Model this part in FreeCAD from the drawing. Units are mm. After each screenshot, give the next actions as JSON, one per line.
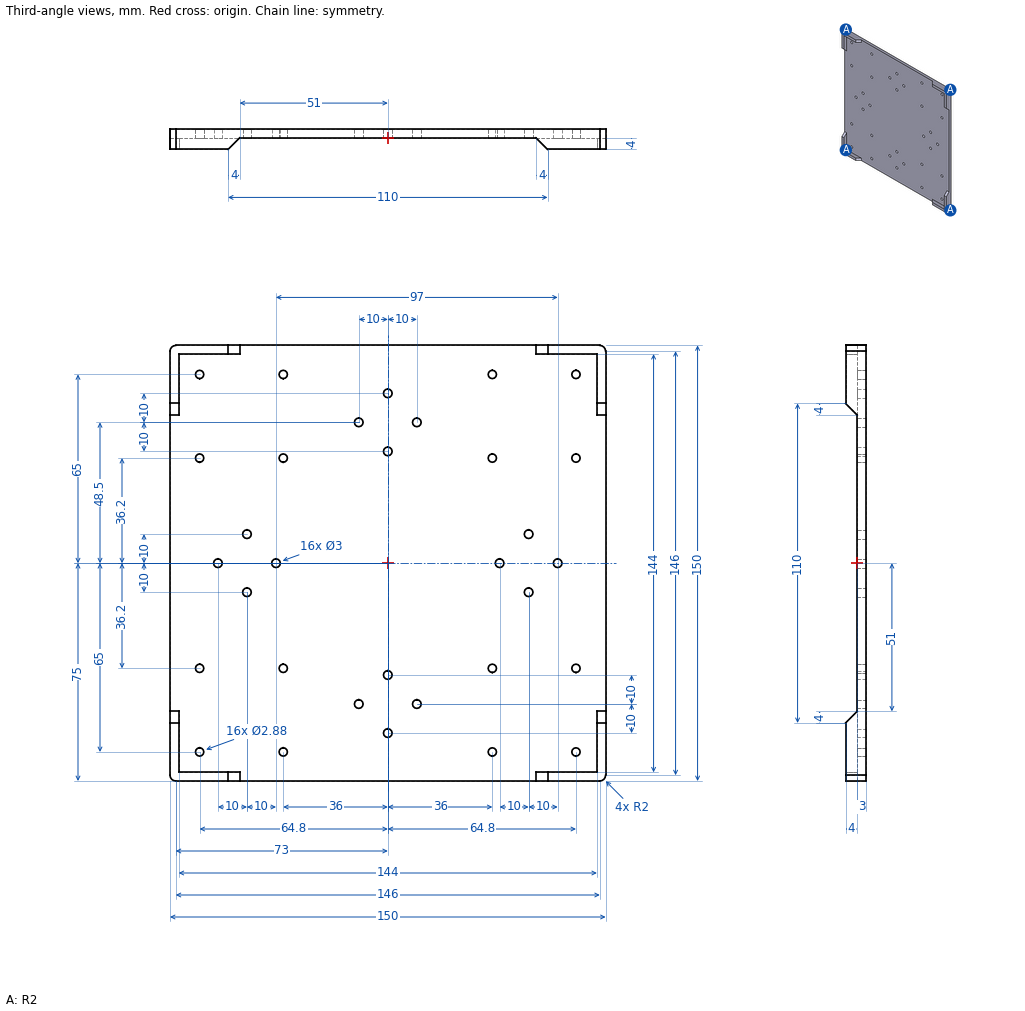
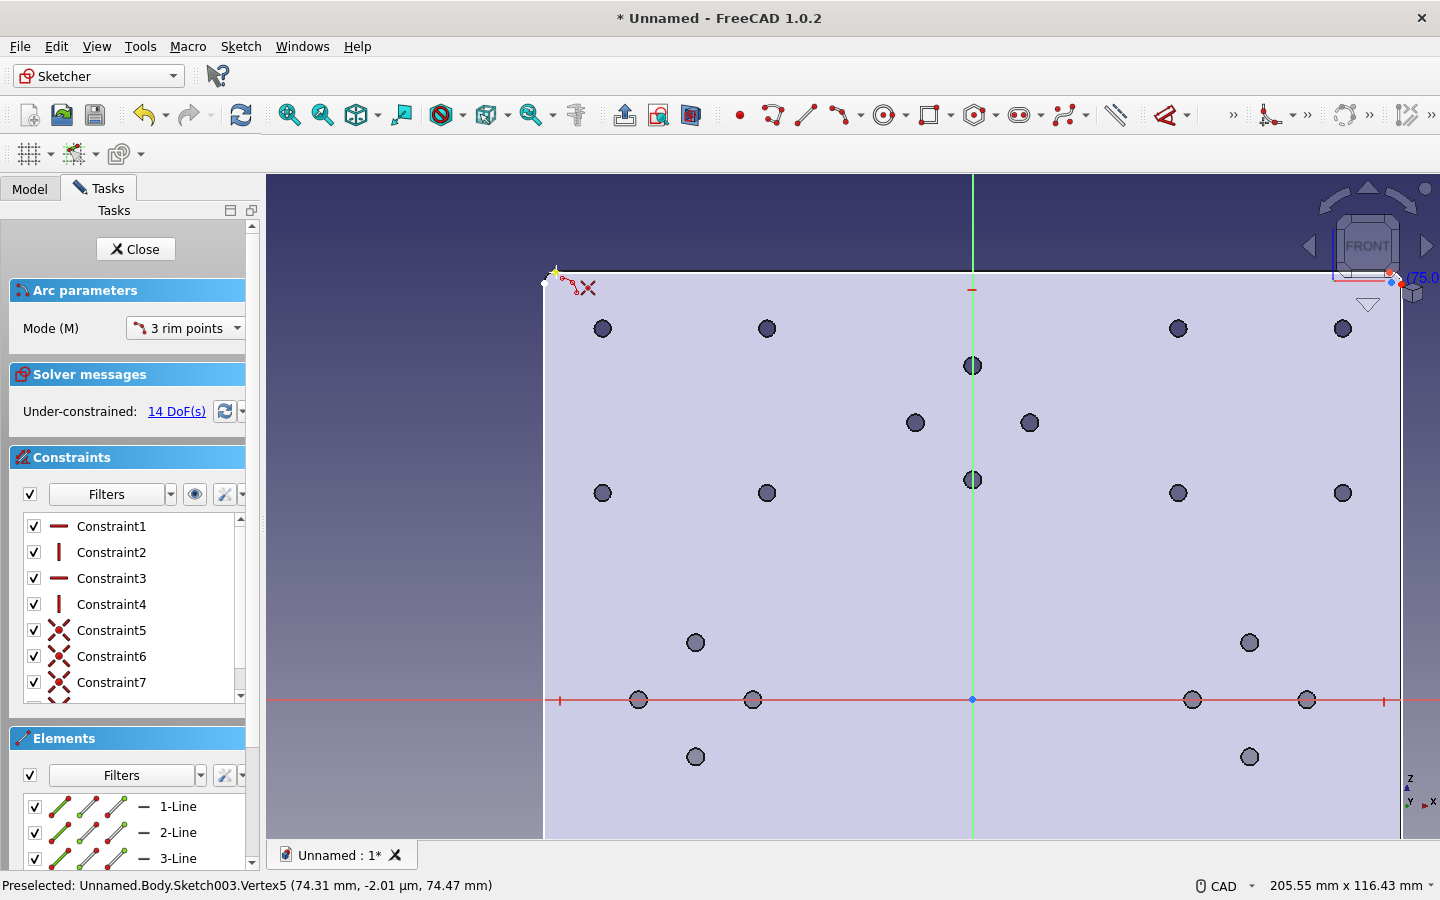
{"action": "left_click", "coordinate": [556, 273]}
{"action": "left_click", "coordinate": [544, 284]}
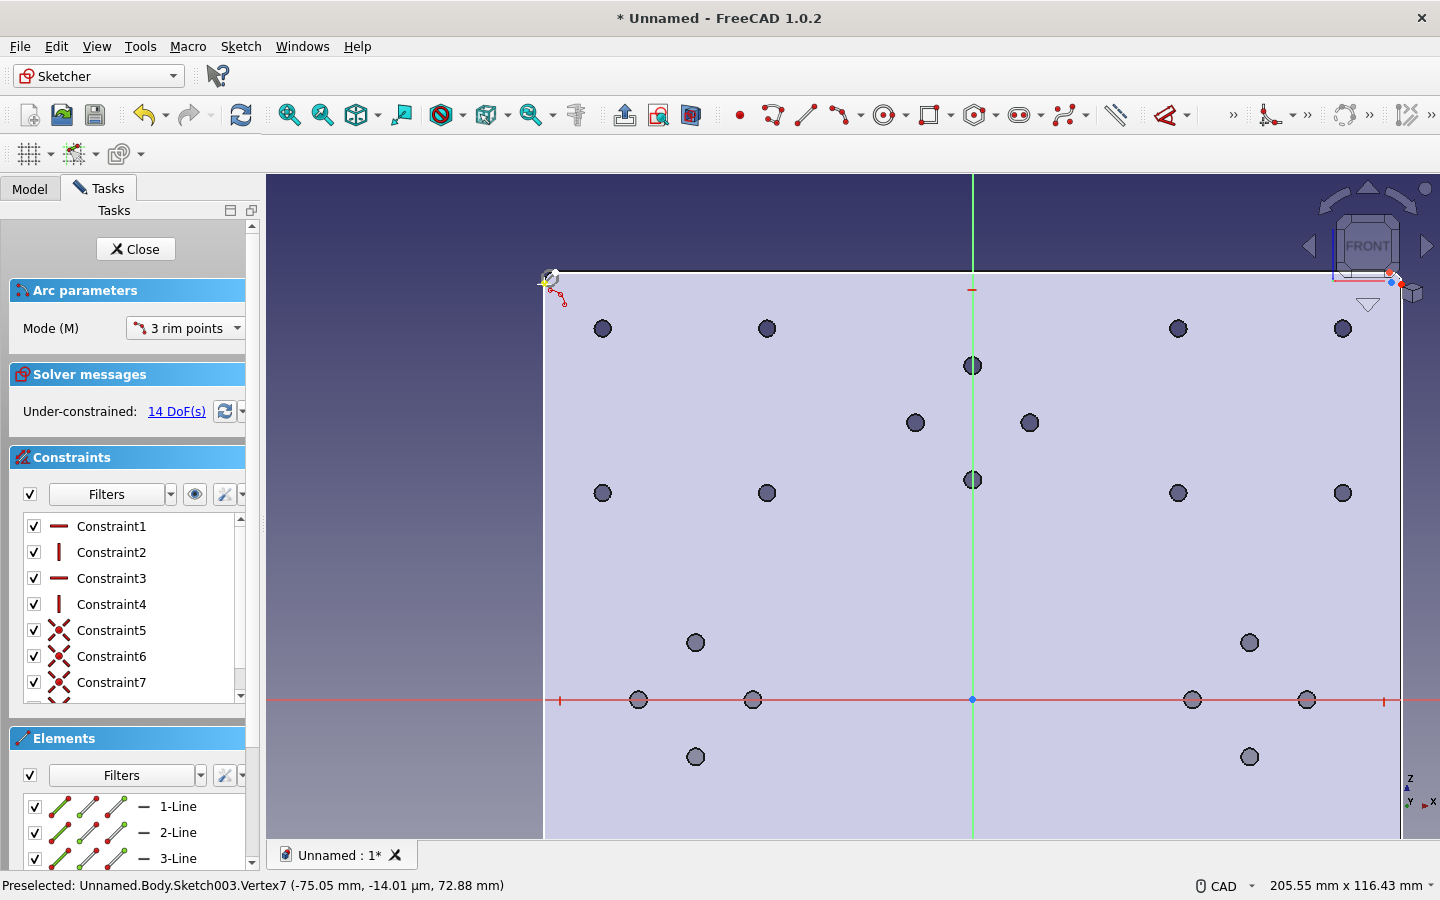
{"action": "scroll", "coordinate": [548, 275], "scroll_direction": "up", "scroll_amount": 8}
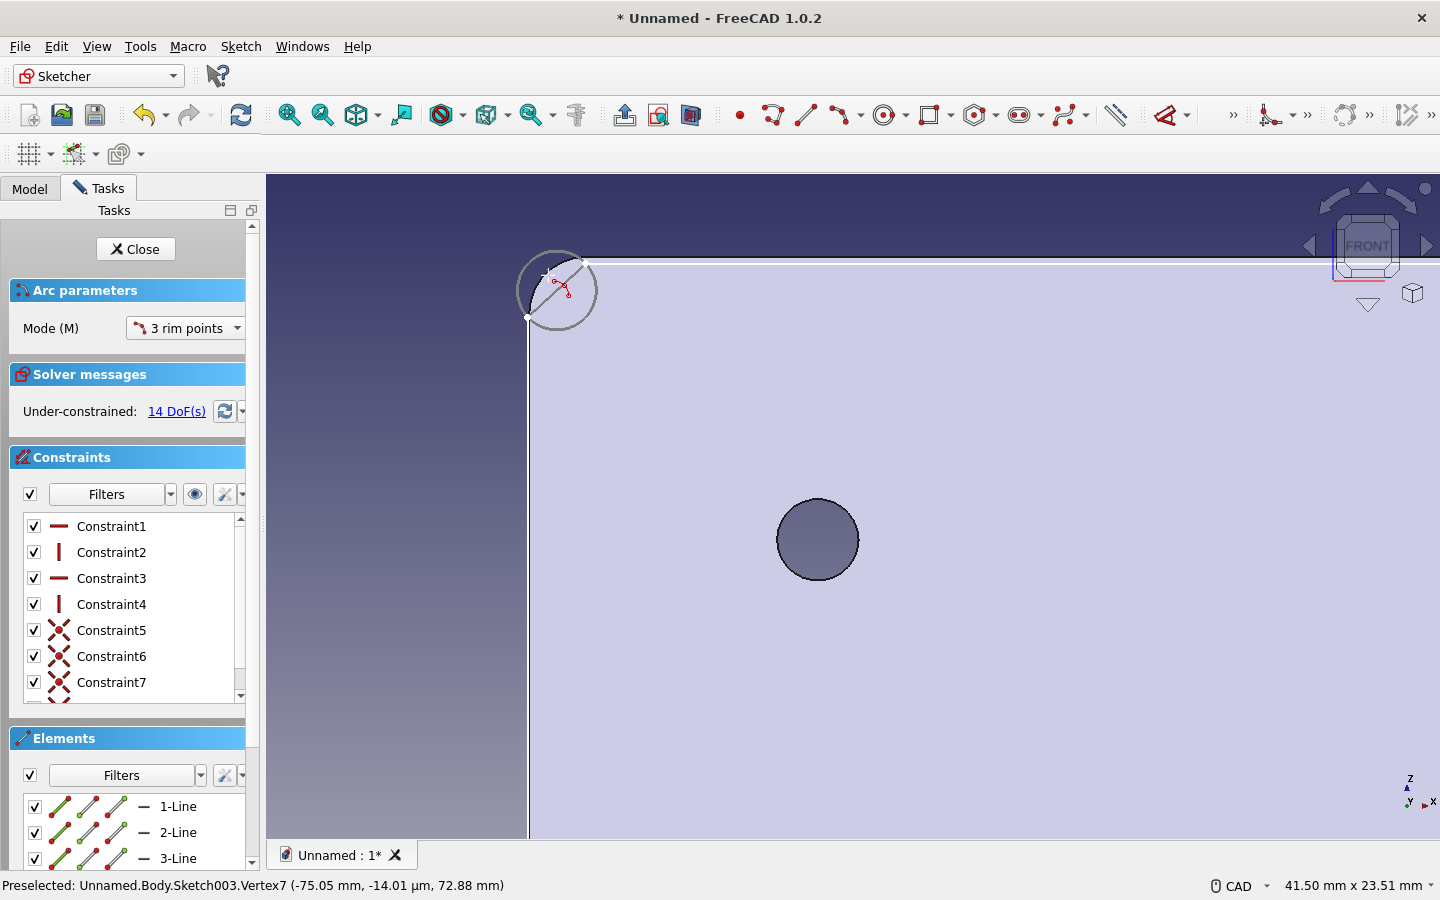
{"action": "left_click", "coordinate": [546, 274]}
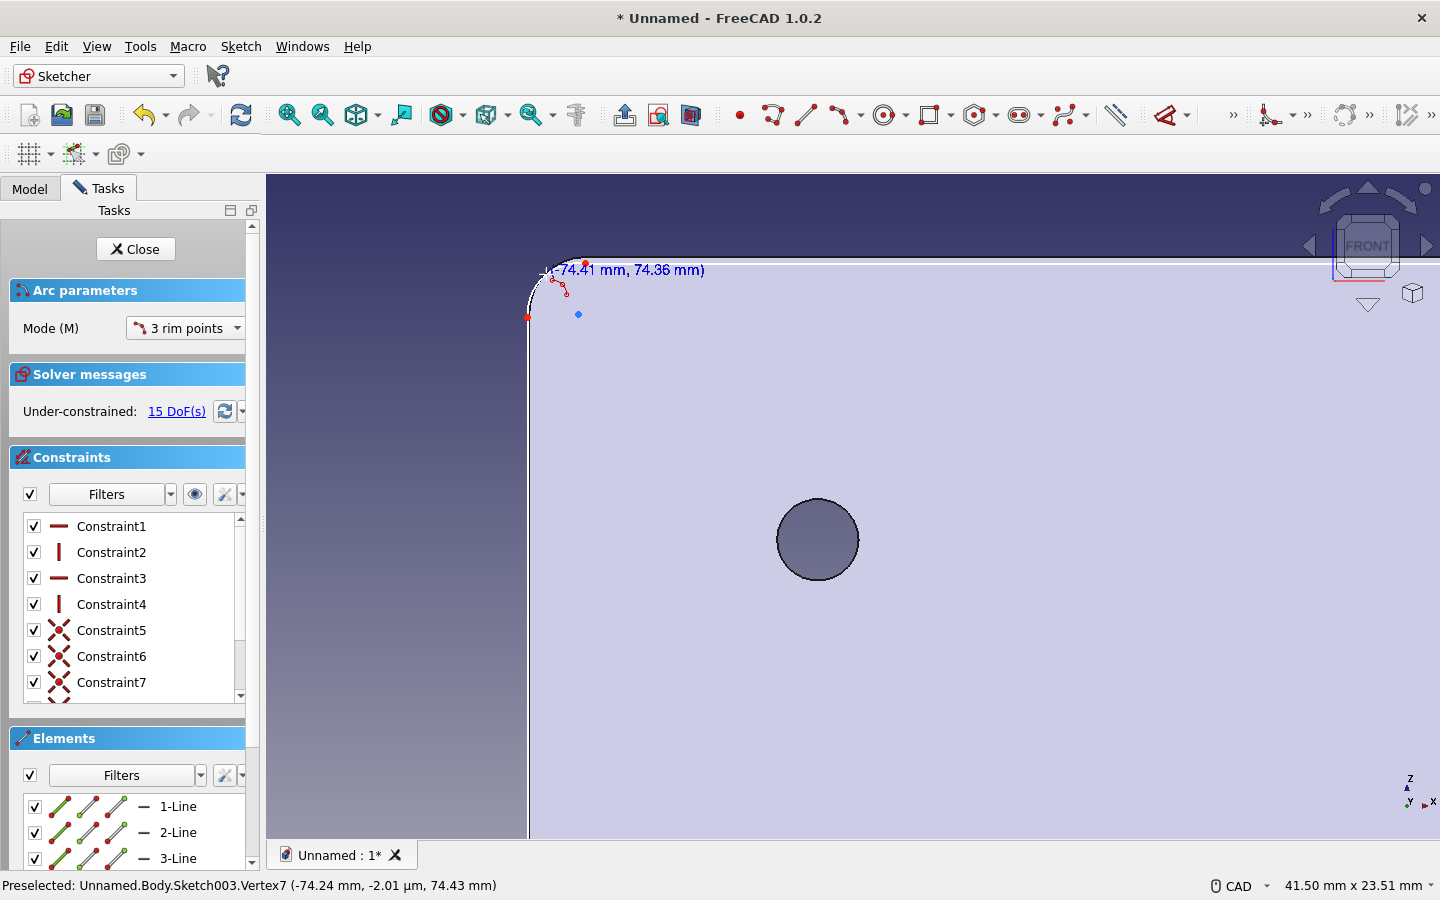
{"action": "scroll", "coordinate": [552, 273], "scroll_direction": "down", "scroll_amount": 11}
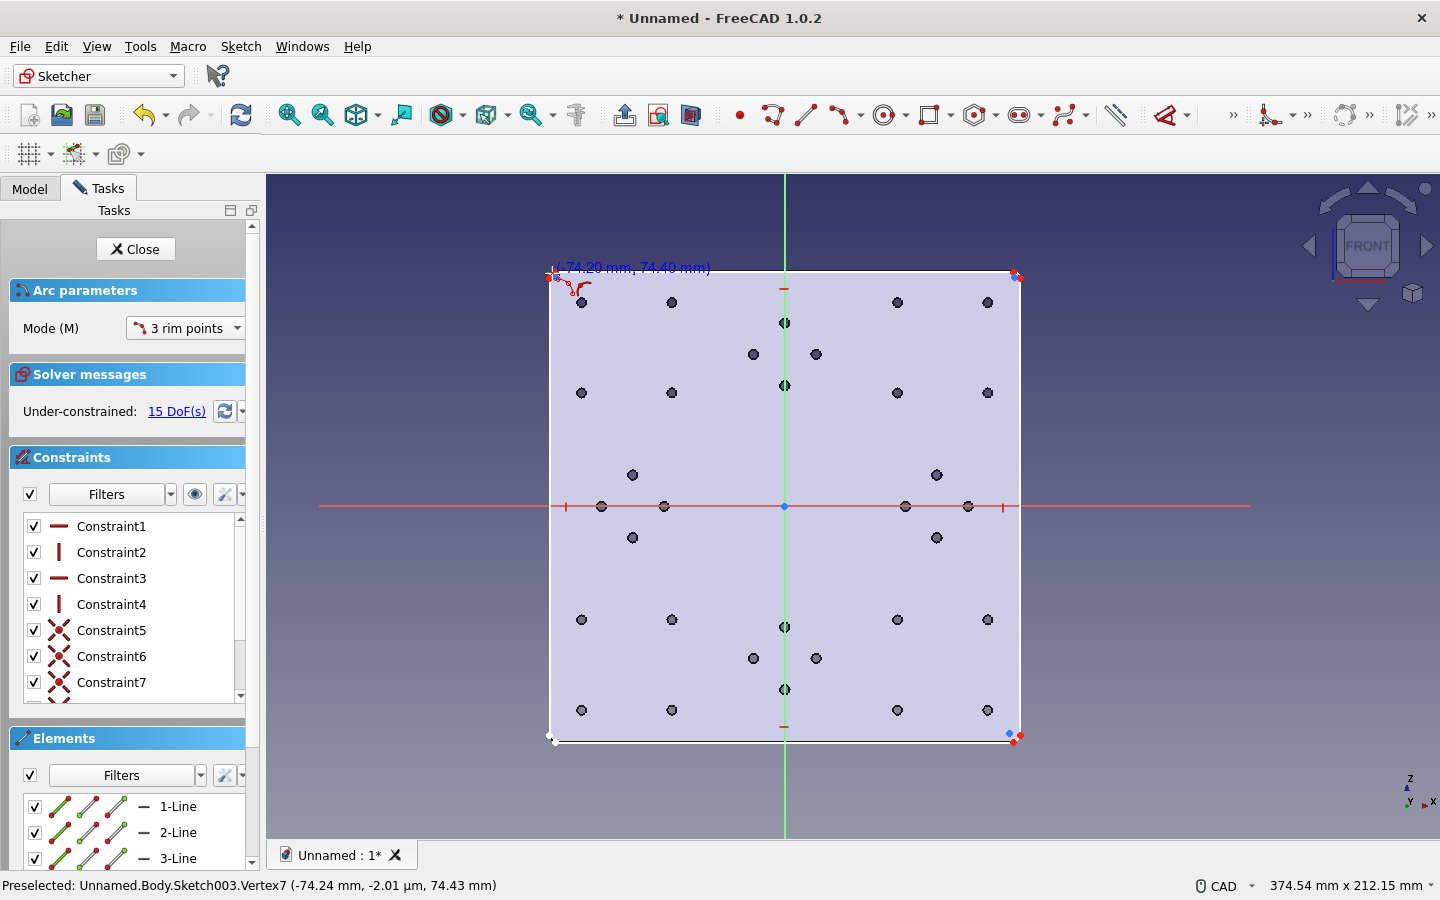
{"action": "scroll", "coordinate": [550, 735], "scroll_direction": "up", "scroll_amount": 3}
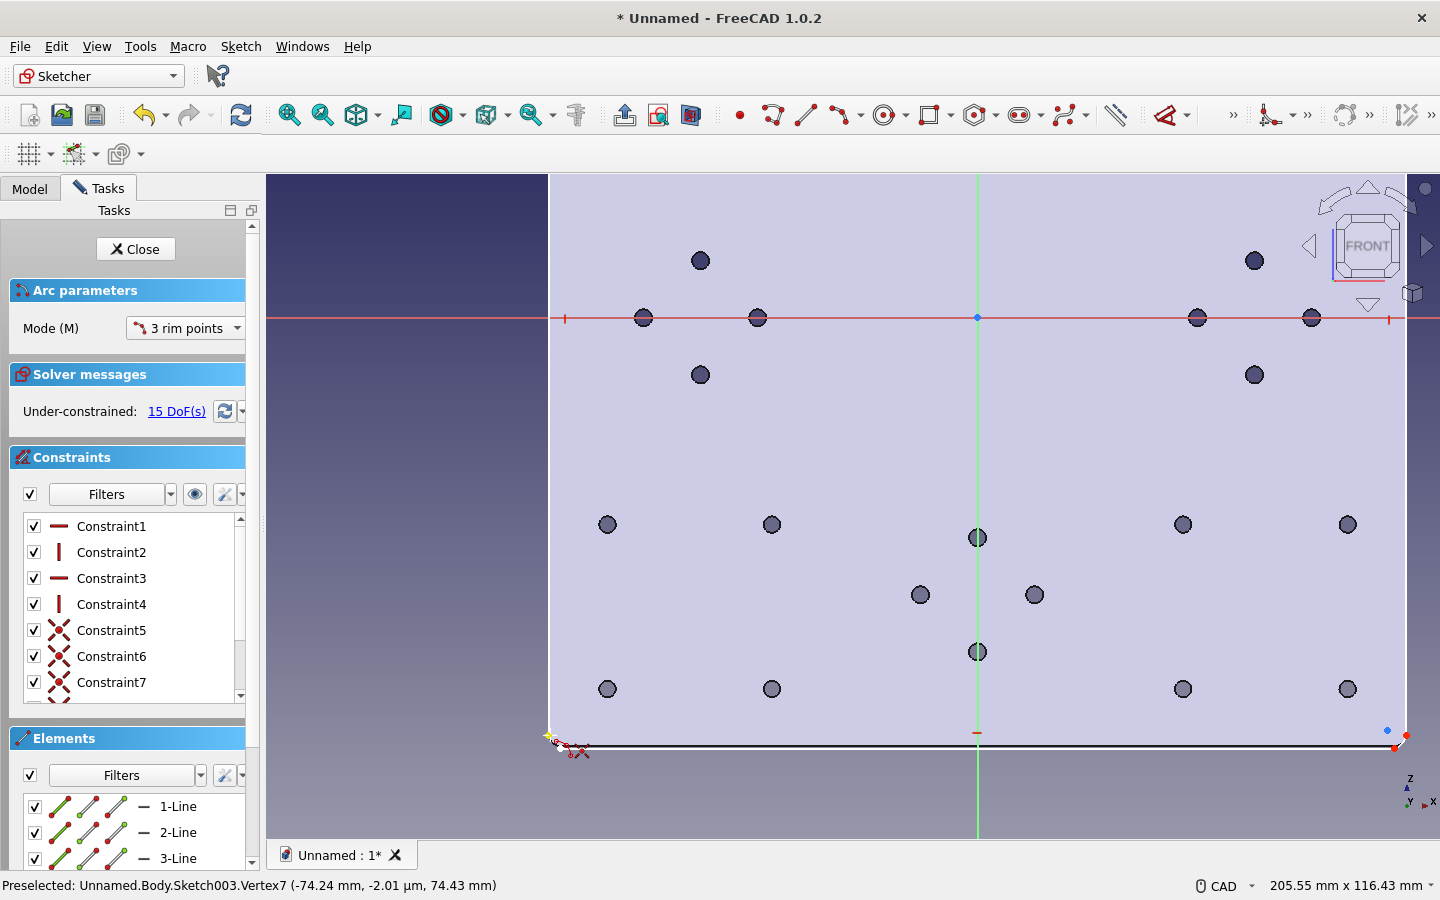
{"action": "left_click", "coordinate": [549, 736]}
{"action": "left_click", "coordinate": [560, 749]}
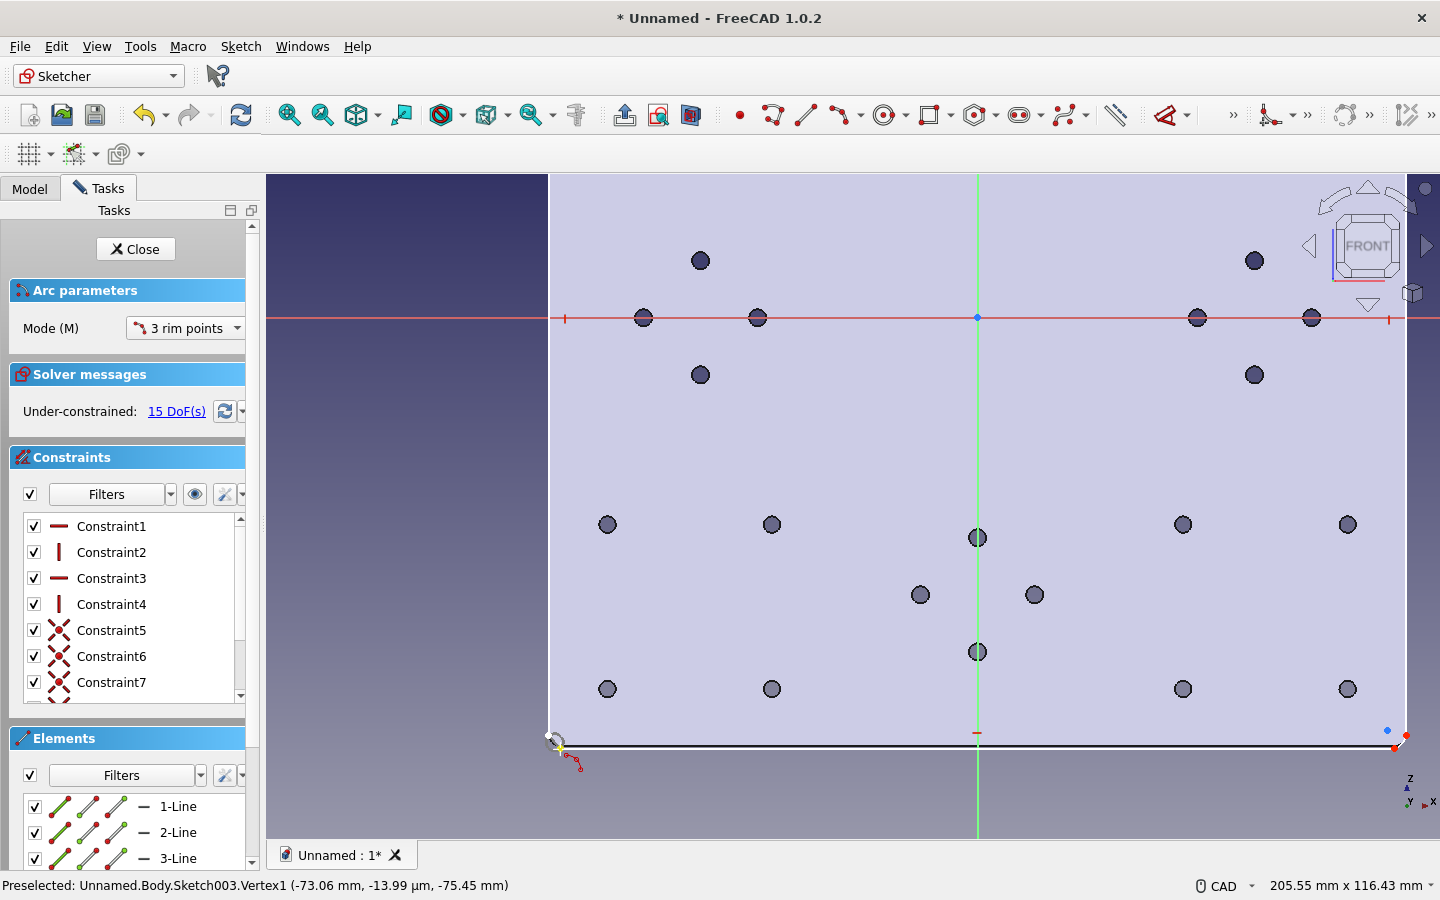
{"action": "scroll", "coordinate": [553, 743], "scroll_direction": "up", "scroll_amount": 8}